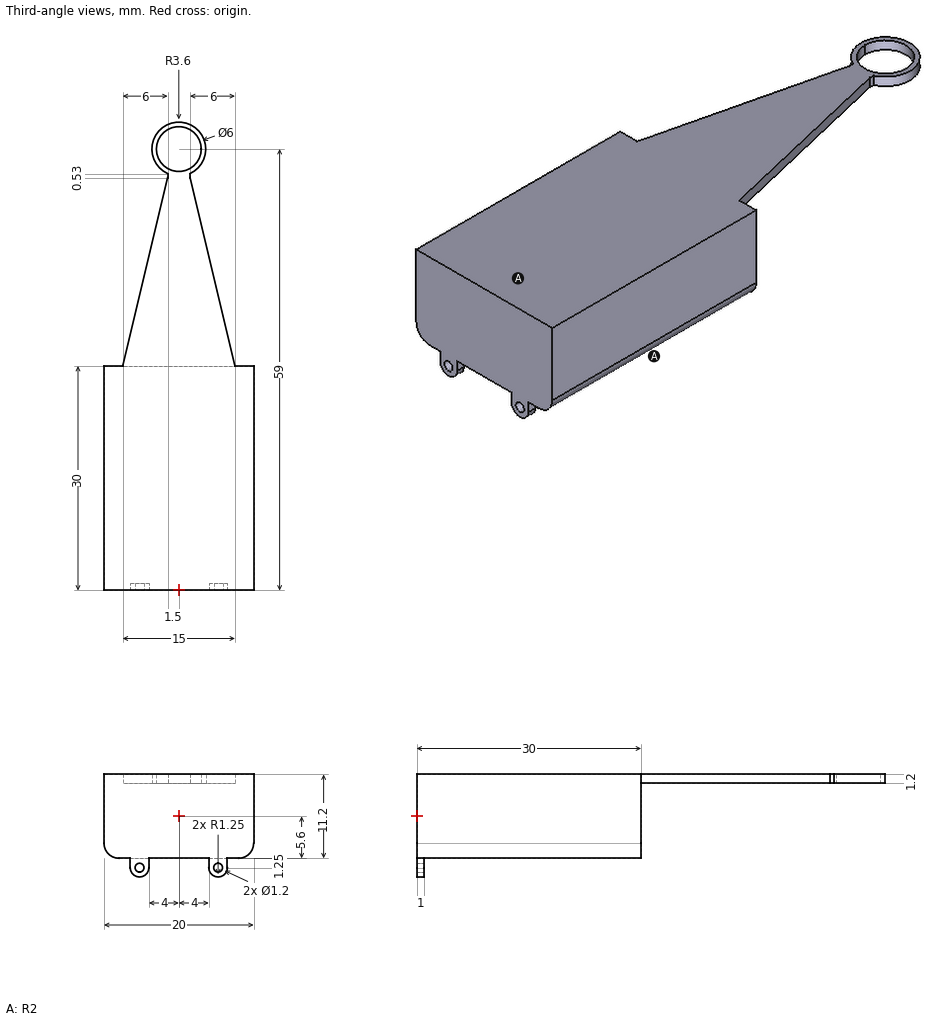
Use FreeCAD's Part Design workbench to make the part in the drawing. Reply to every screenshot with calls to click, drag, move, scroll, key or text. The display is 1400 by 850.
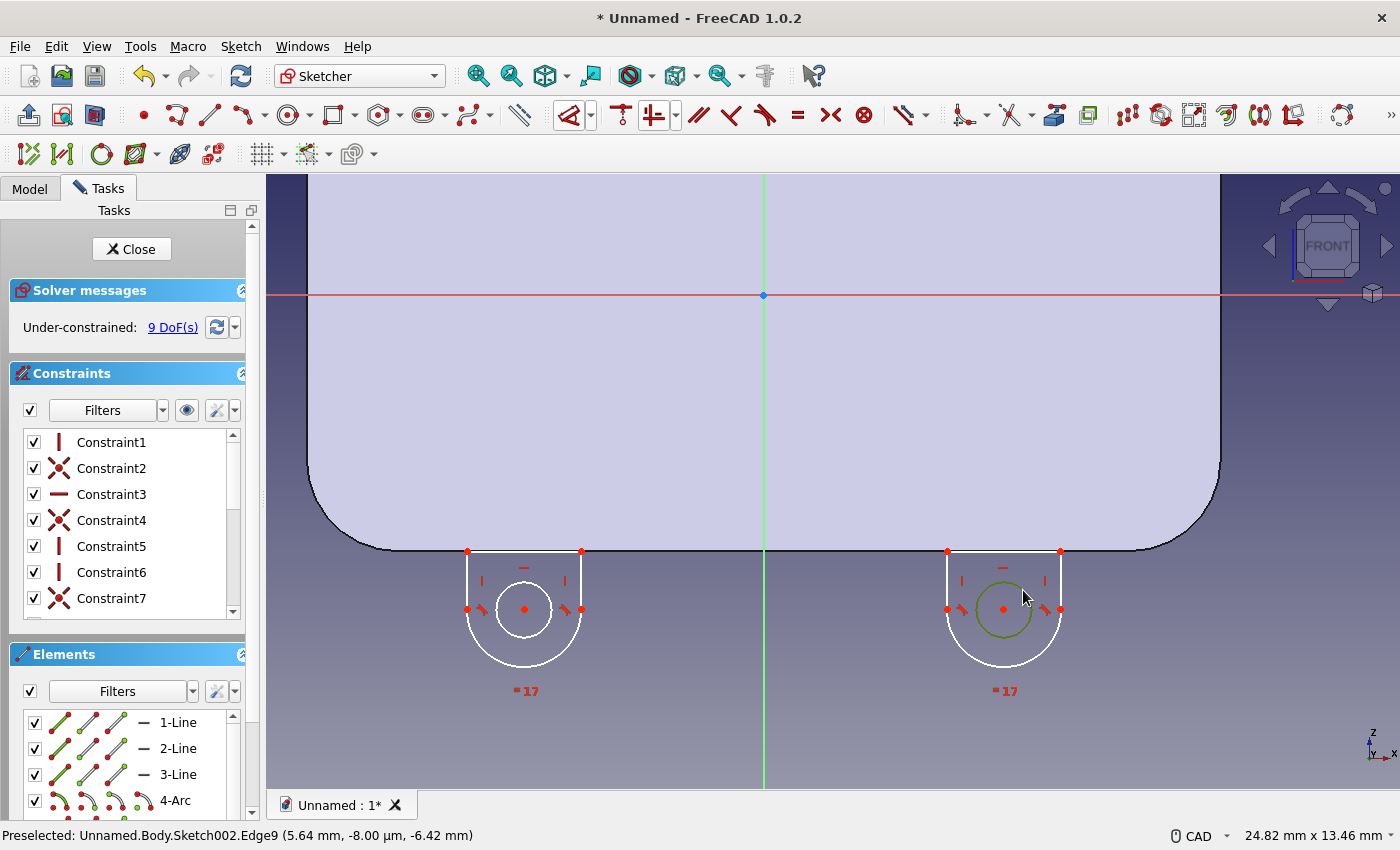
click(543, 590)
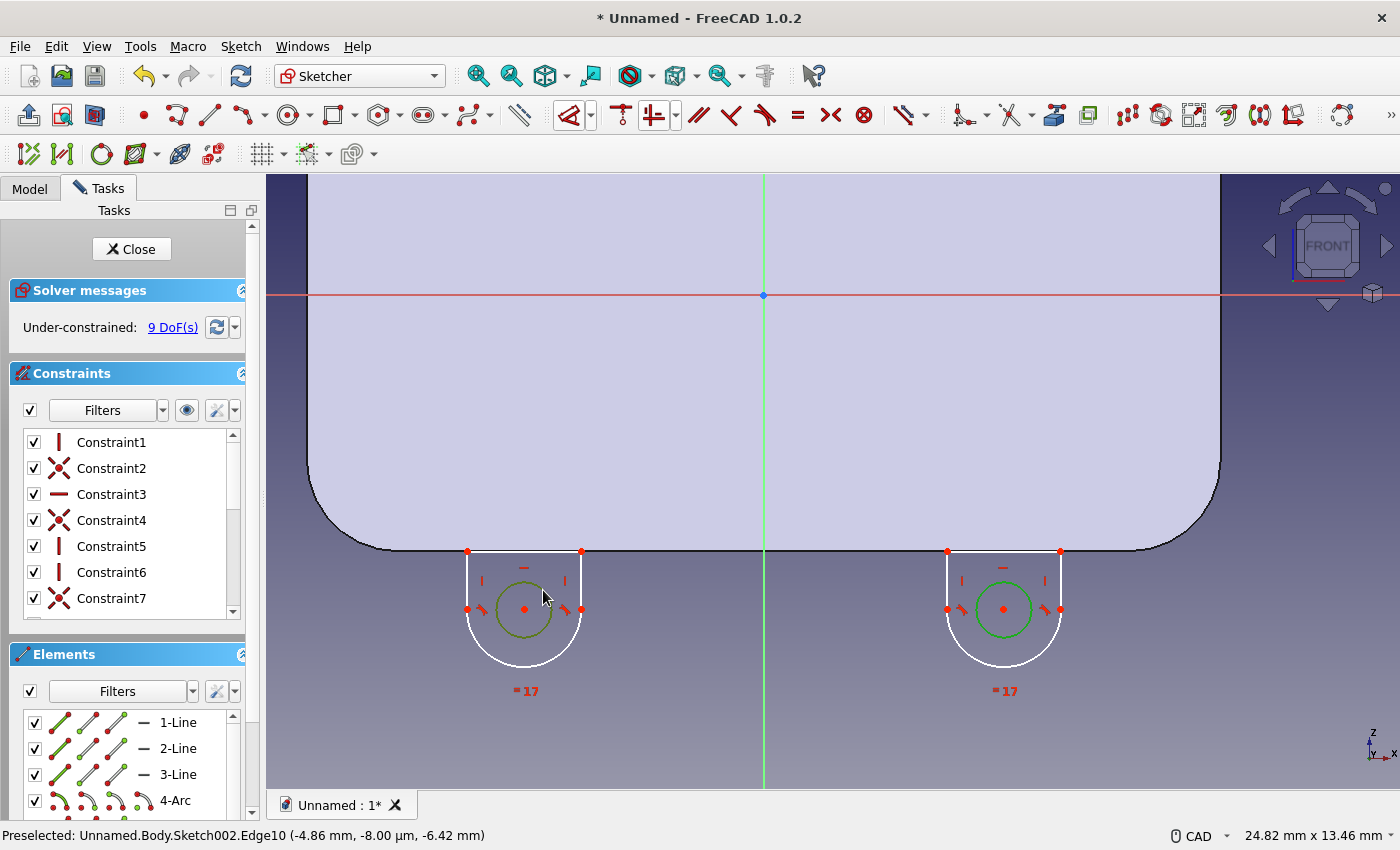
key(e)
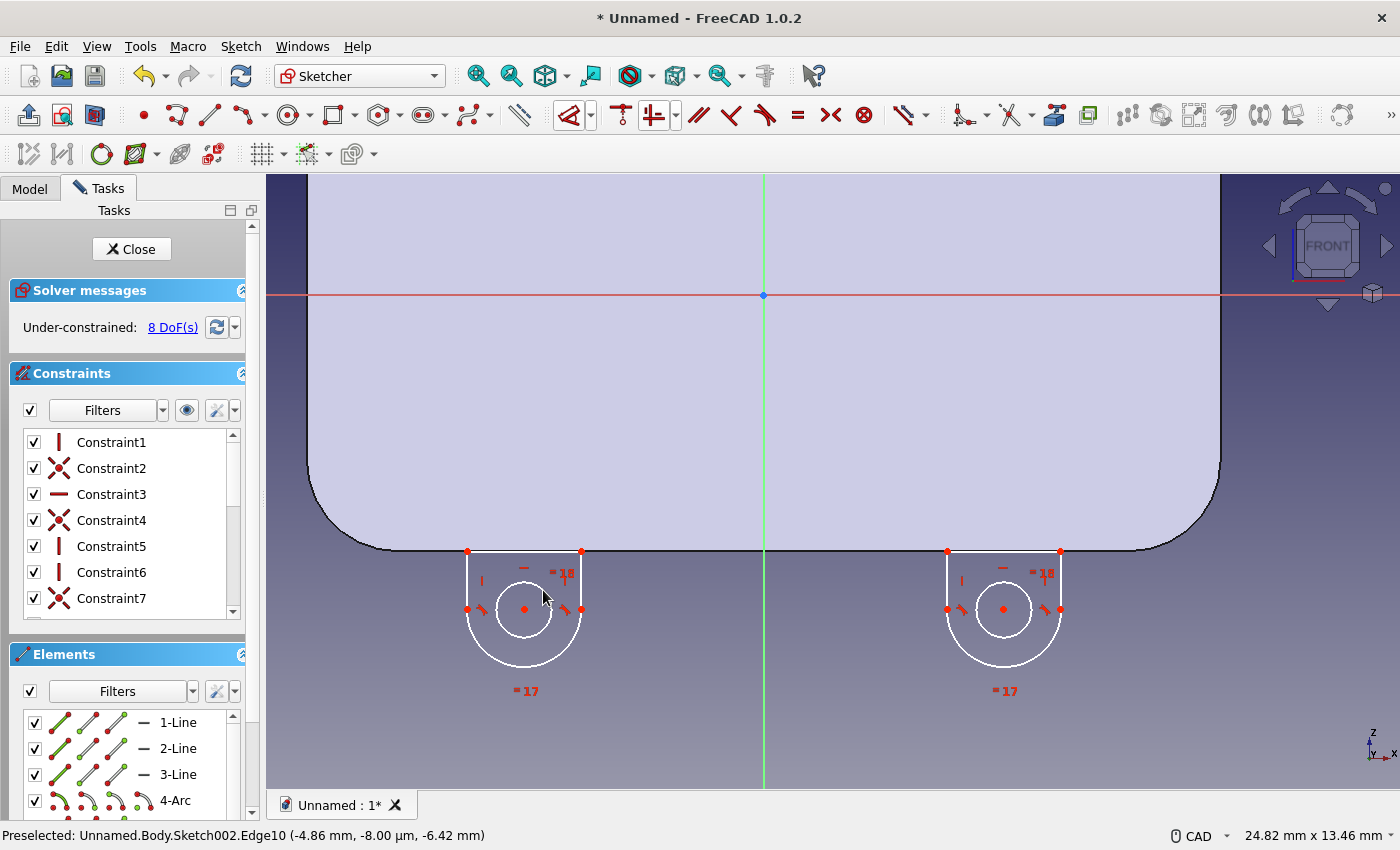
key(d)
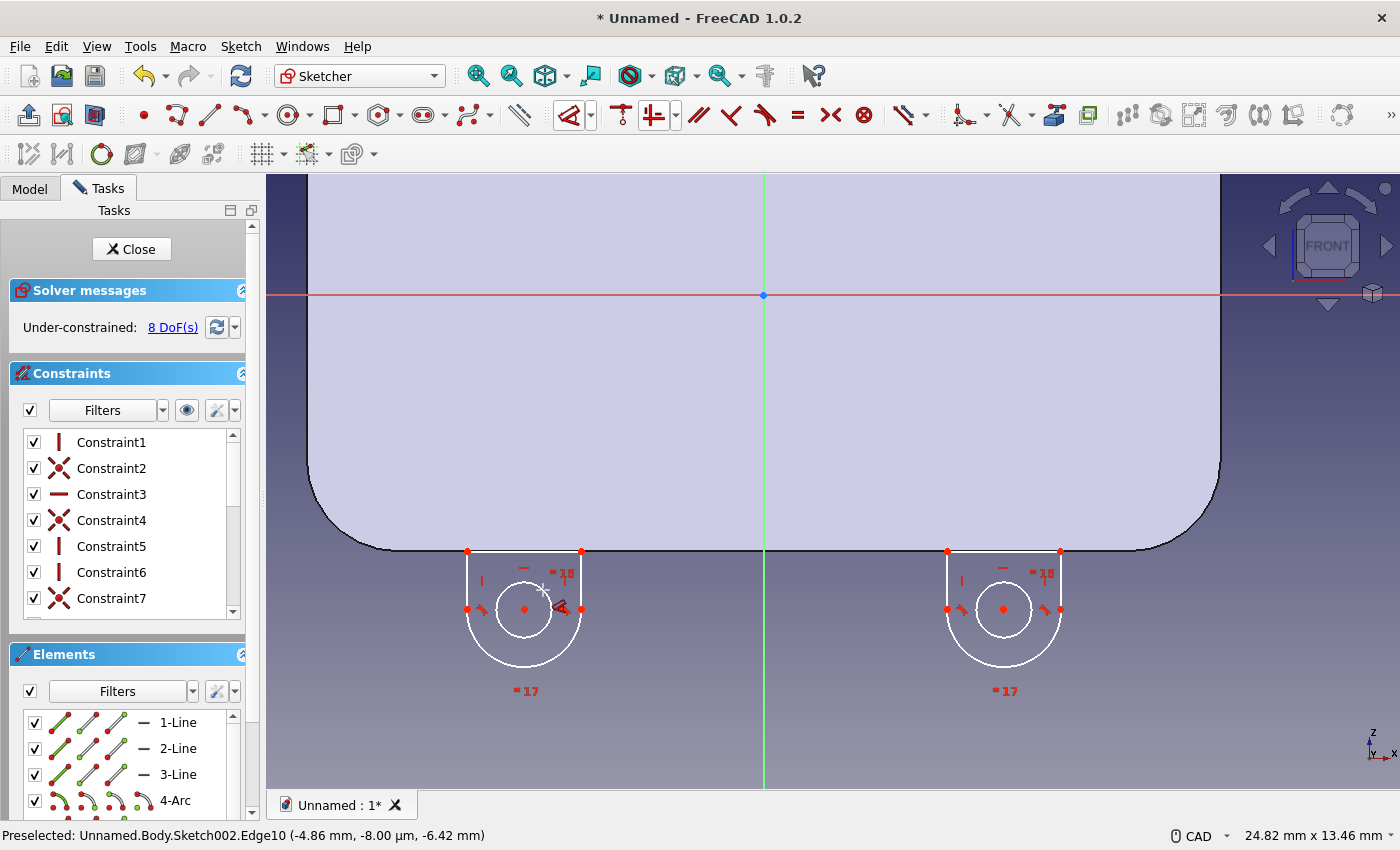
click(970, 656)
click(951, 682)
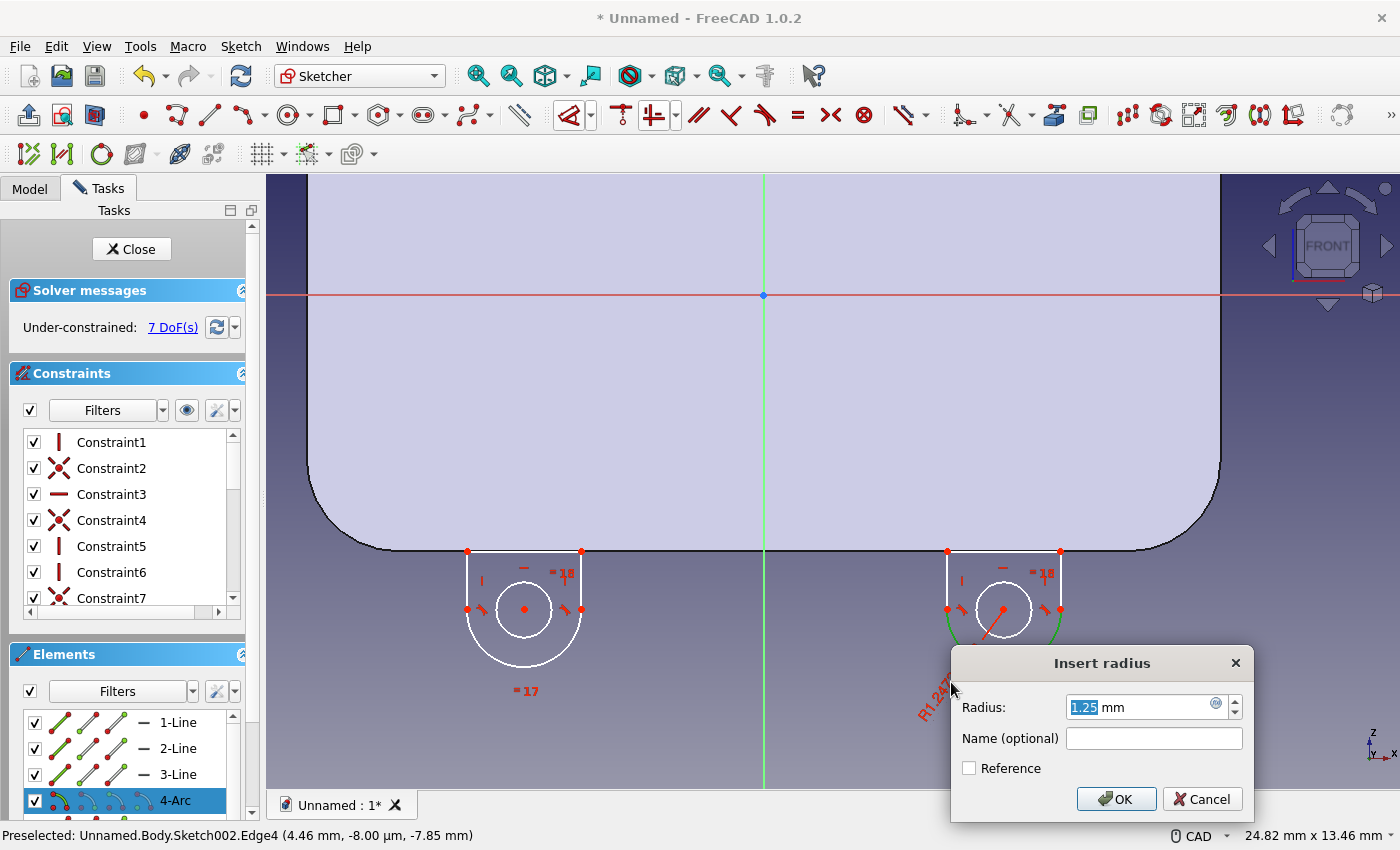
text(1.25)
key(Return)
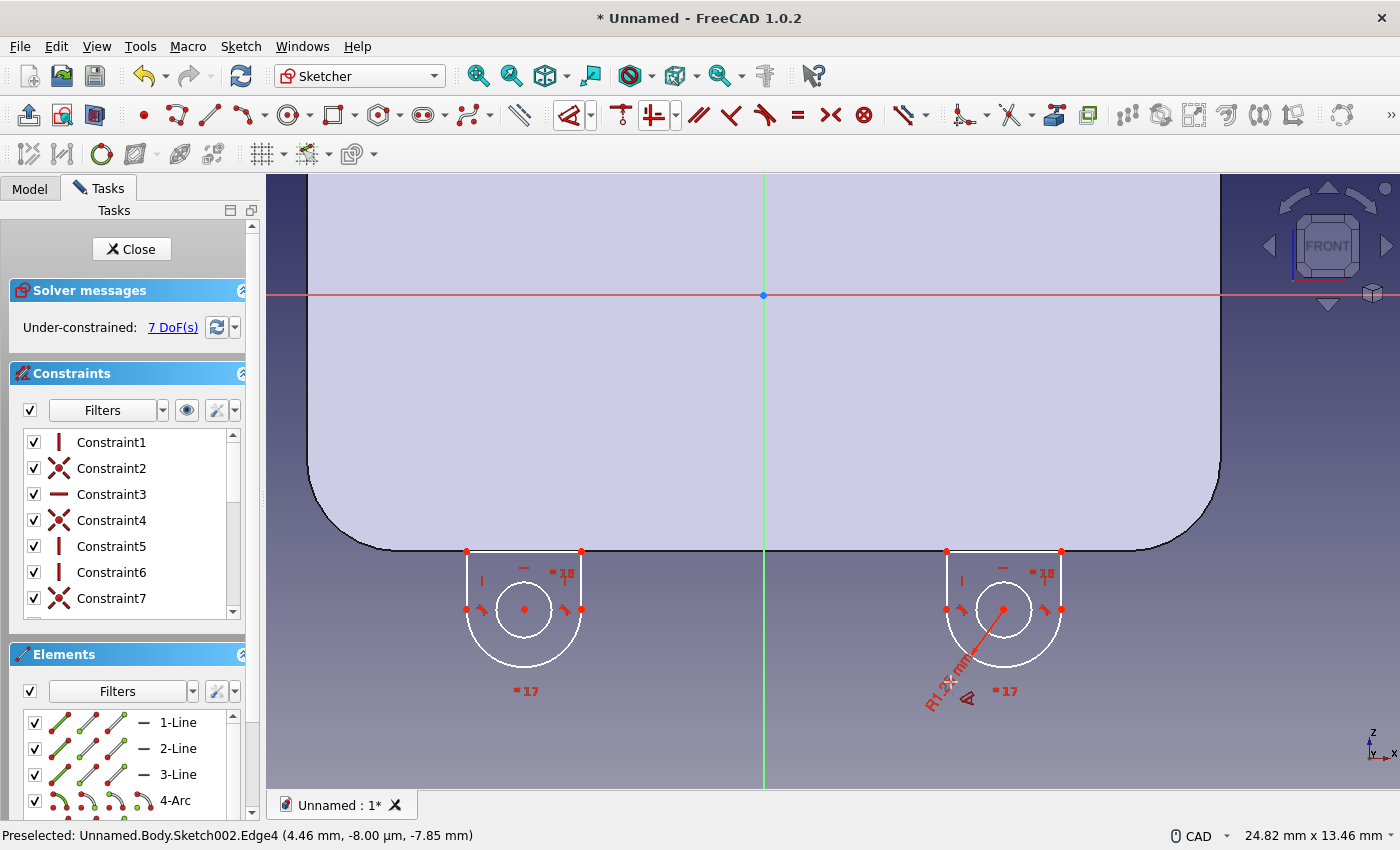
click(1023, 590)
click(1045, 567)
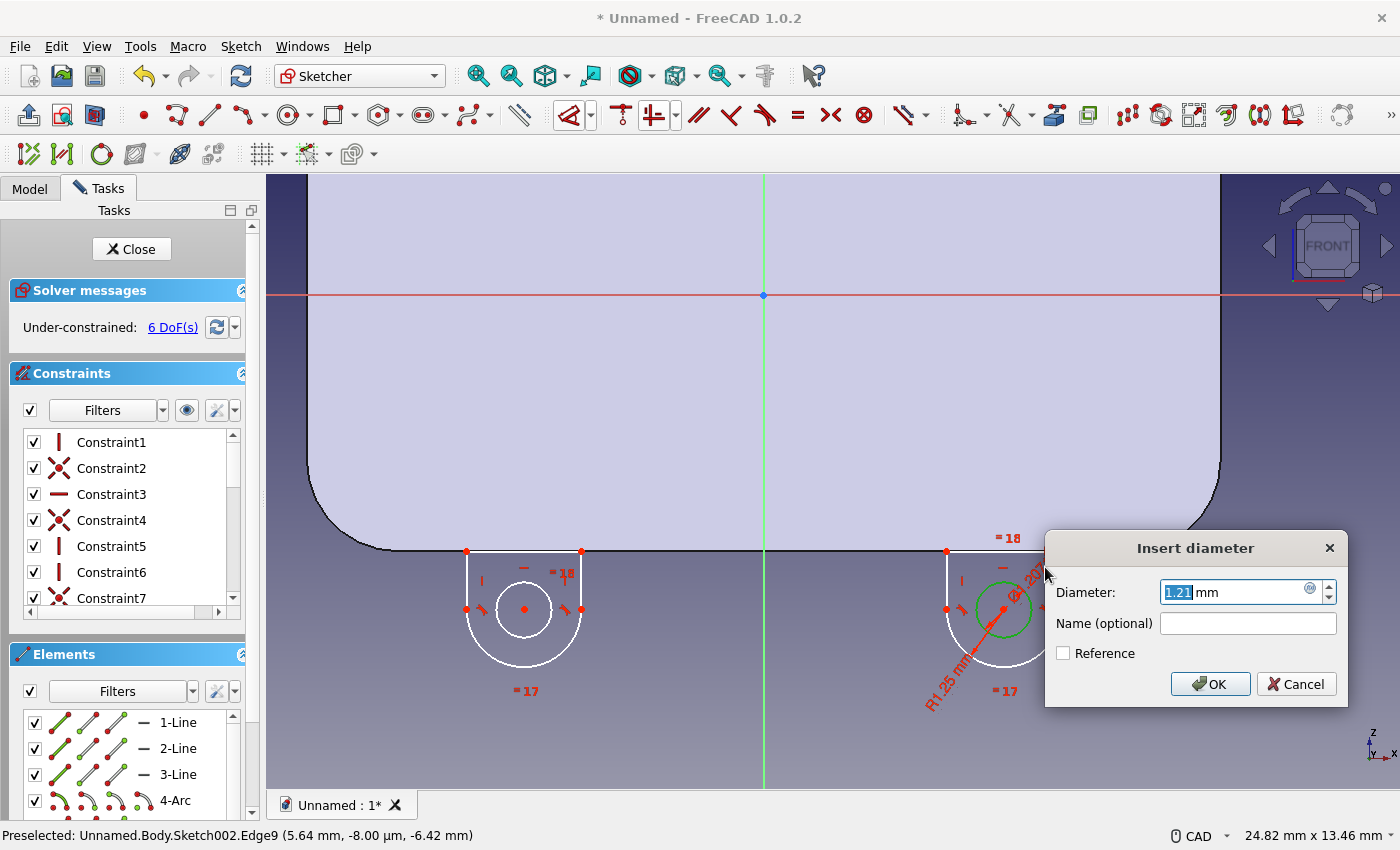
text(1.2)
key(Return)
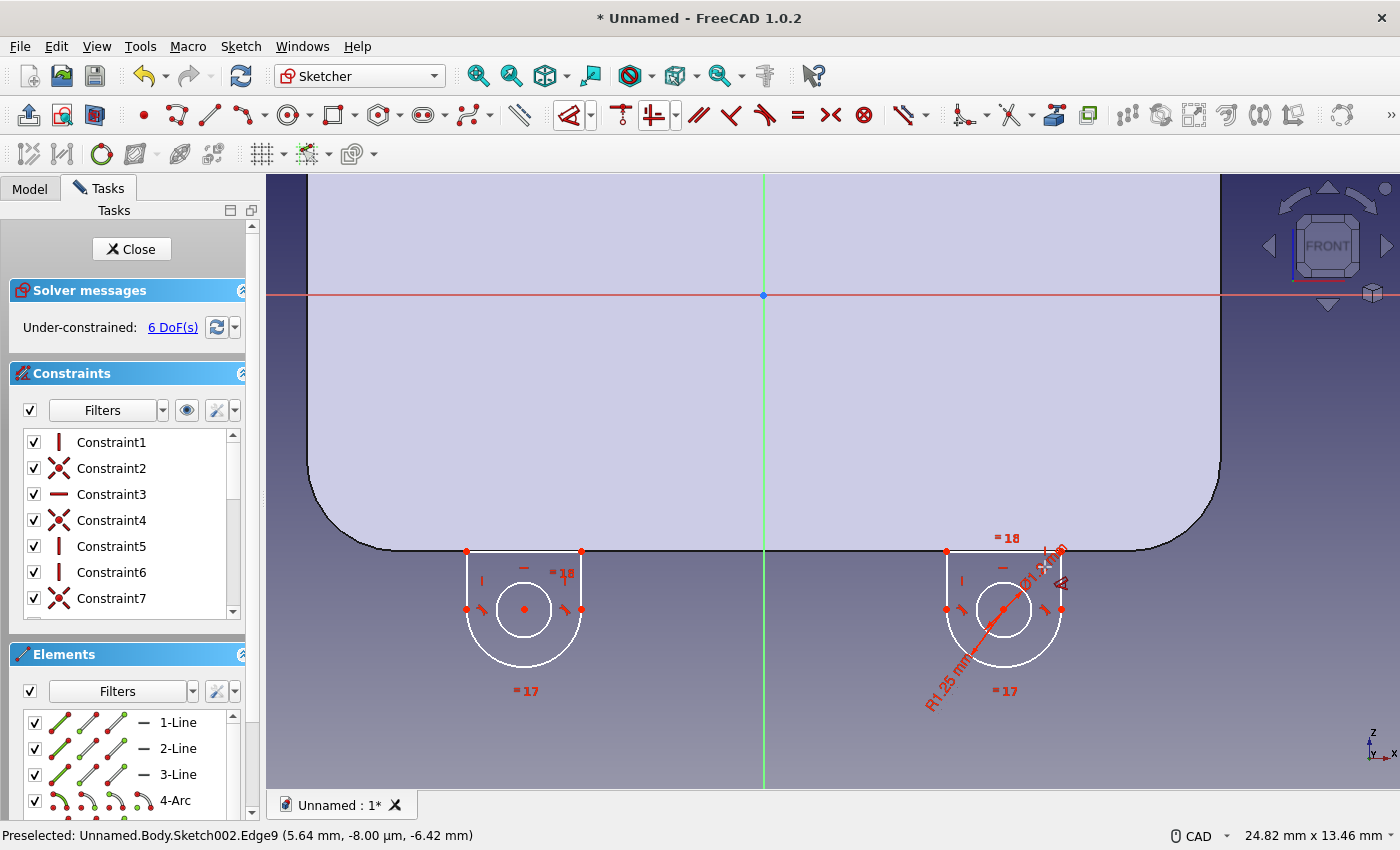
click(947, 552)
click(855, 261)